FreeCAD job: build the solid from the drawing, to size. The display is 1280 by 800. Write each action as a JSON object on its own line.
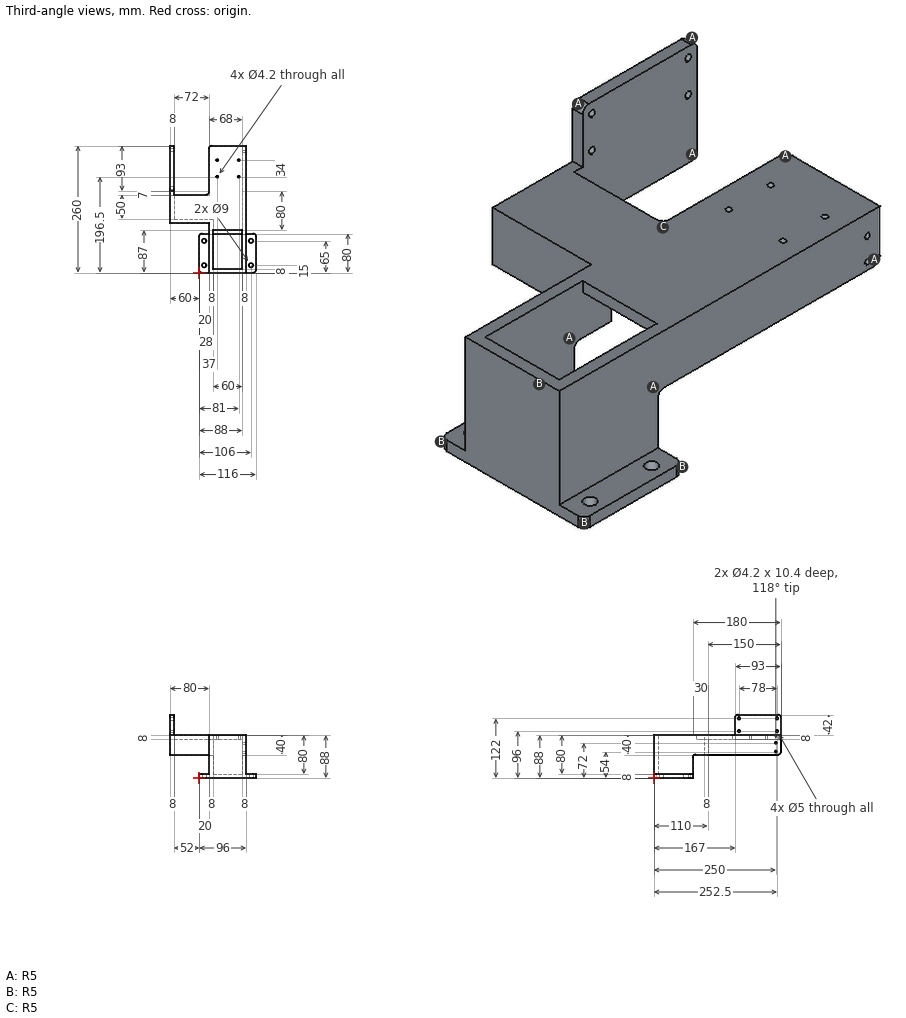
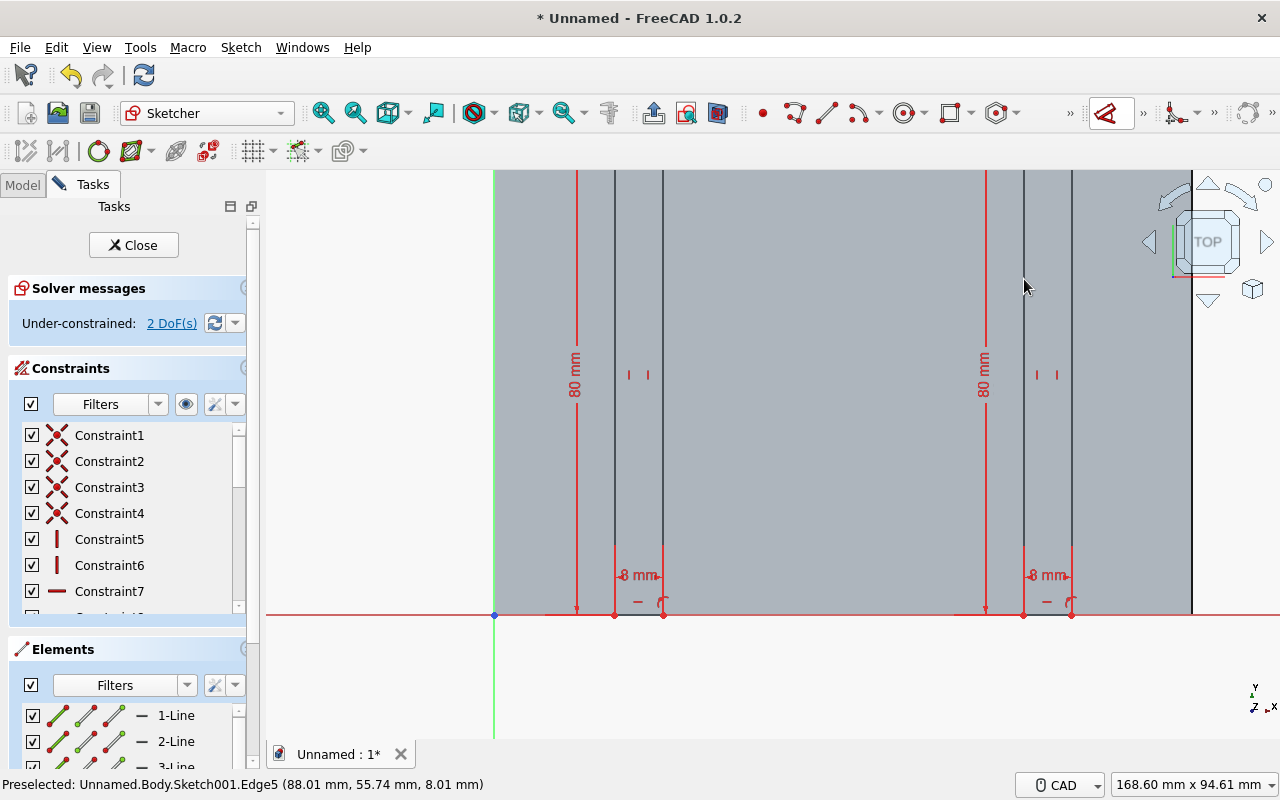
{"action": "scroll", "coordinate": [350, 711], "scroll_direction": "down", "scroll_amount": 1}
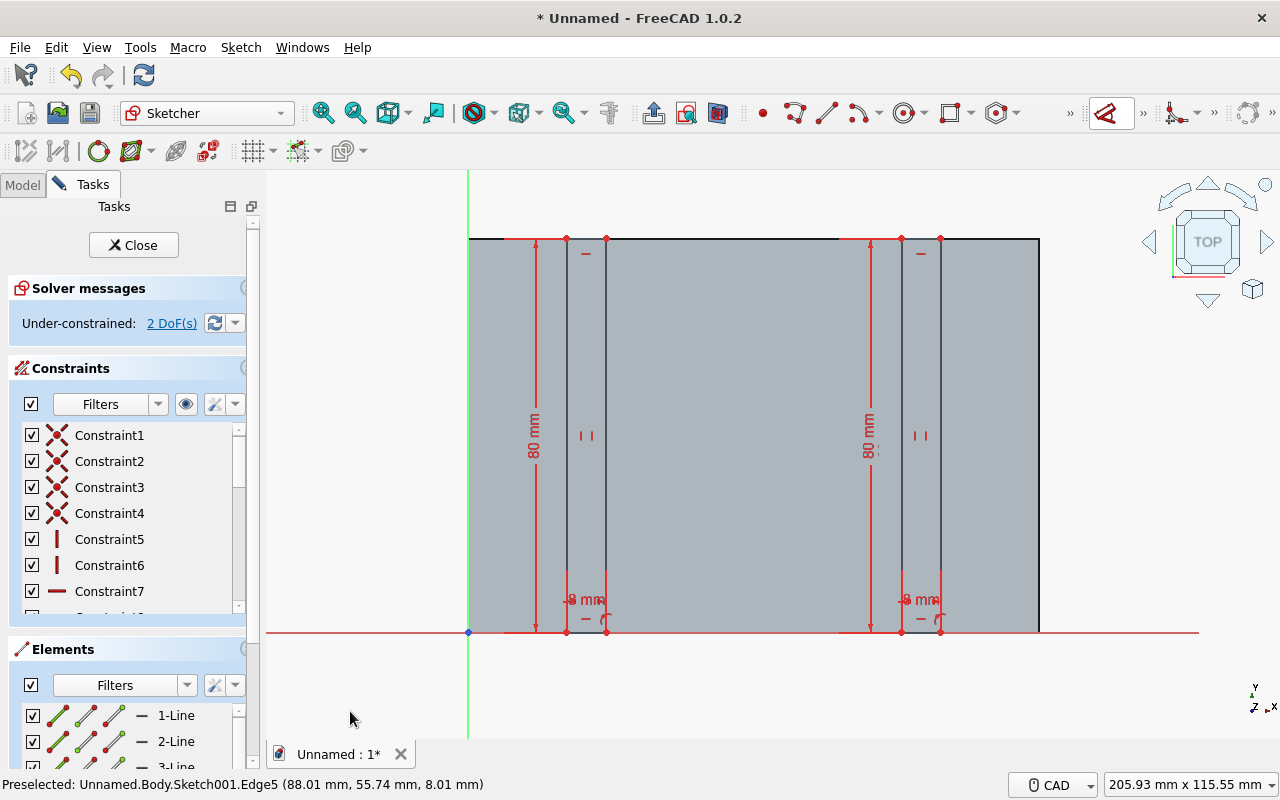
{"action": "left_click", "coordinate": [567, 239]}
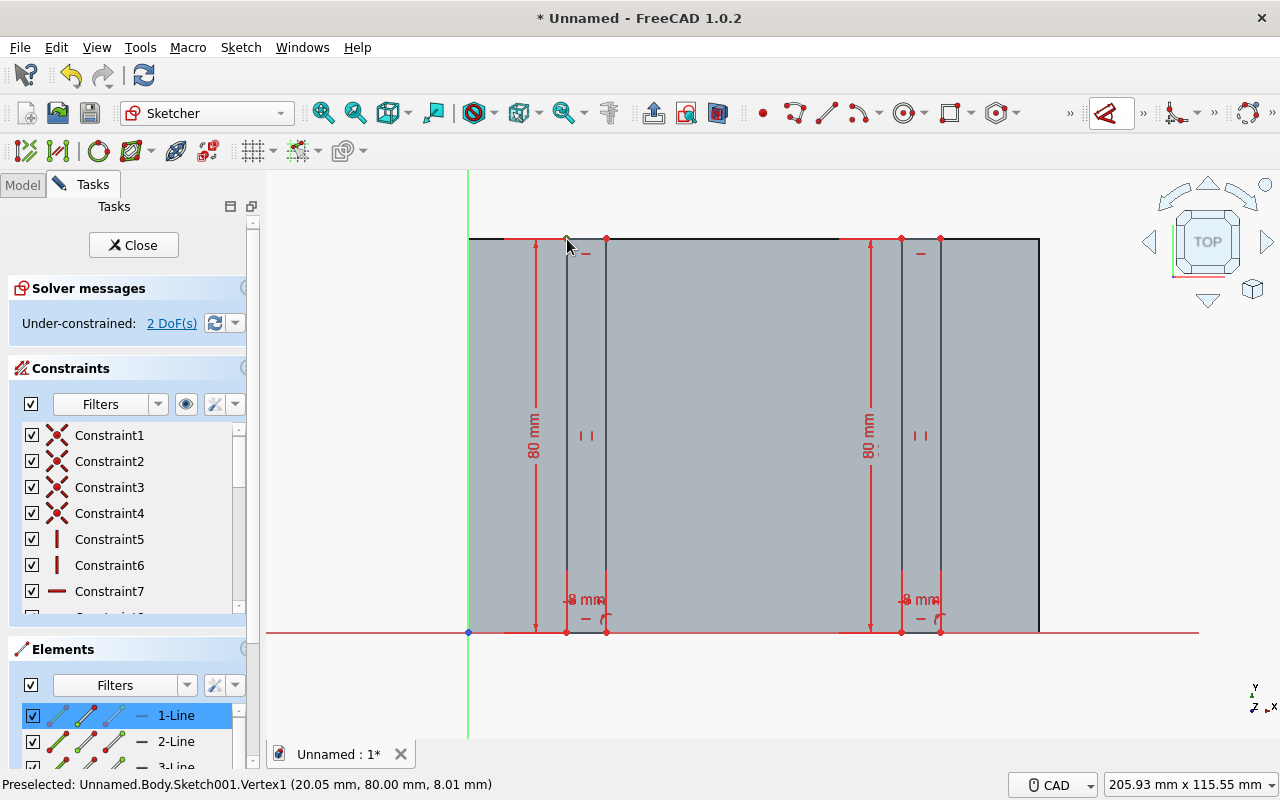
{"action": "left_click", "coordinate": [1128, 114]}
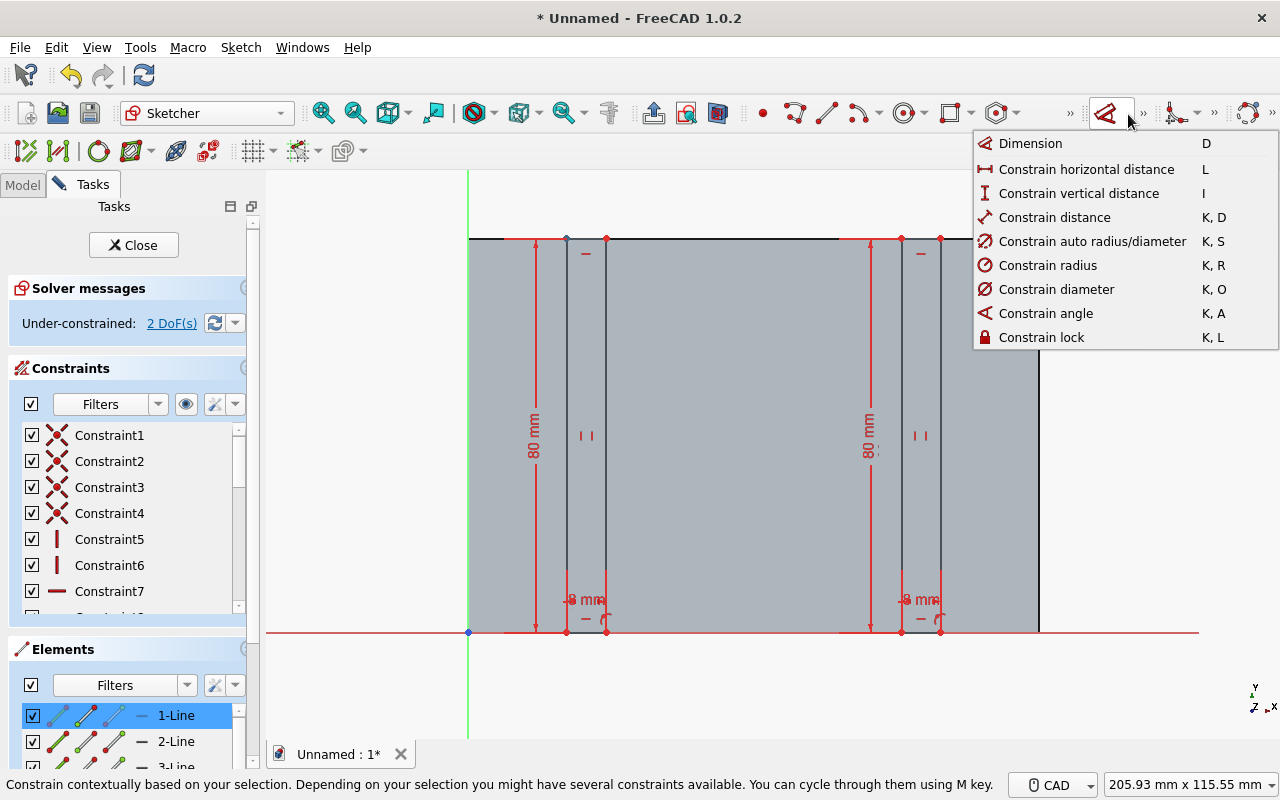
{"action": "left_click", "coordinate": [1126, 169]}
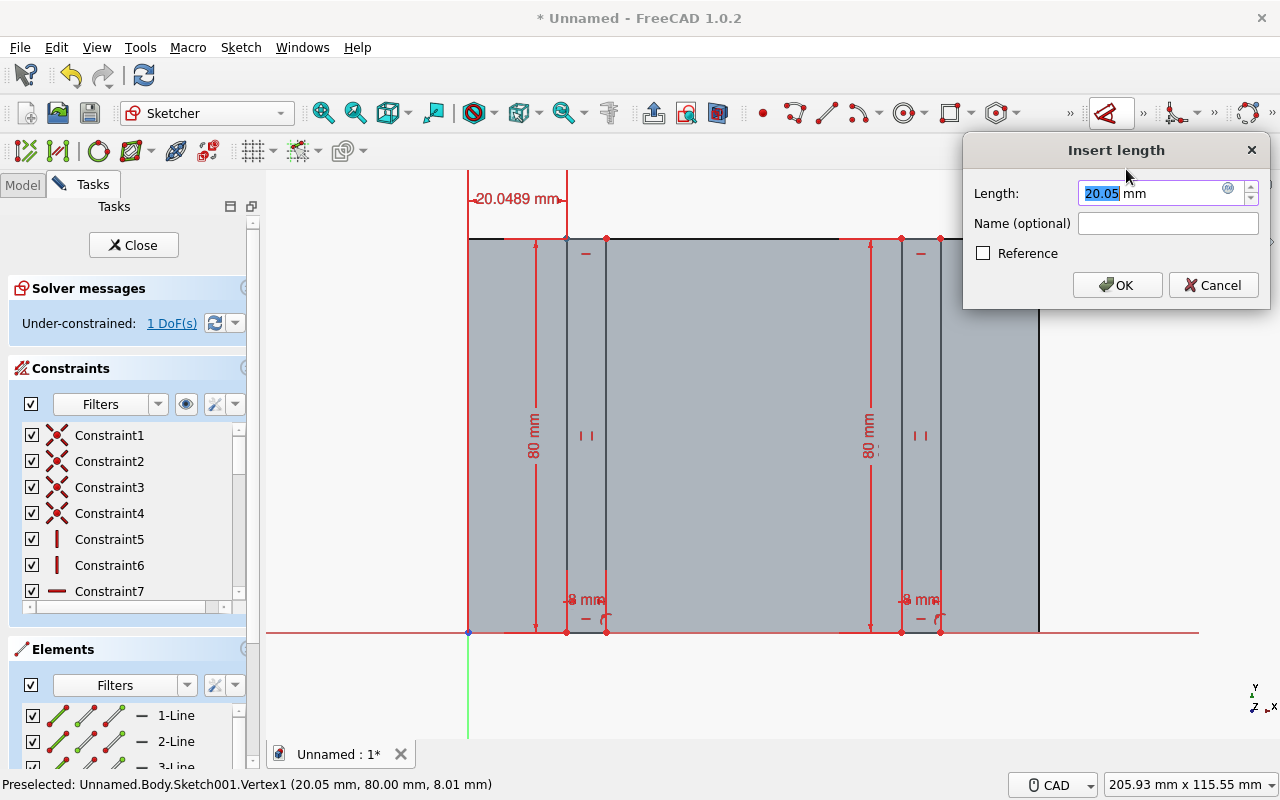
{"action": "type", "text": "20"}
{"action": "key", "text": "Return"}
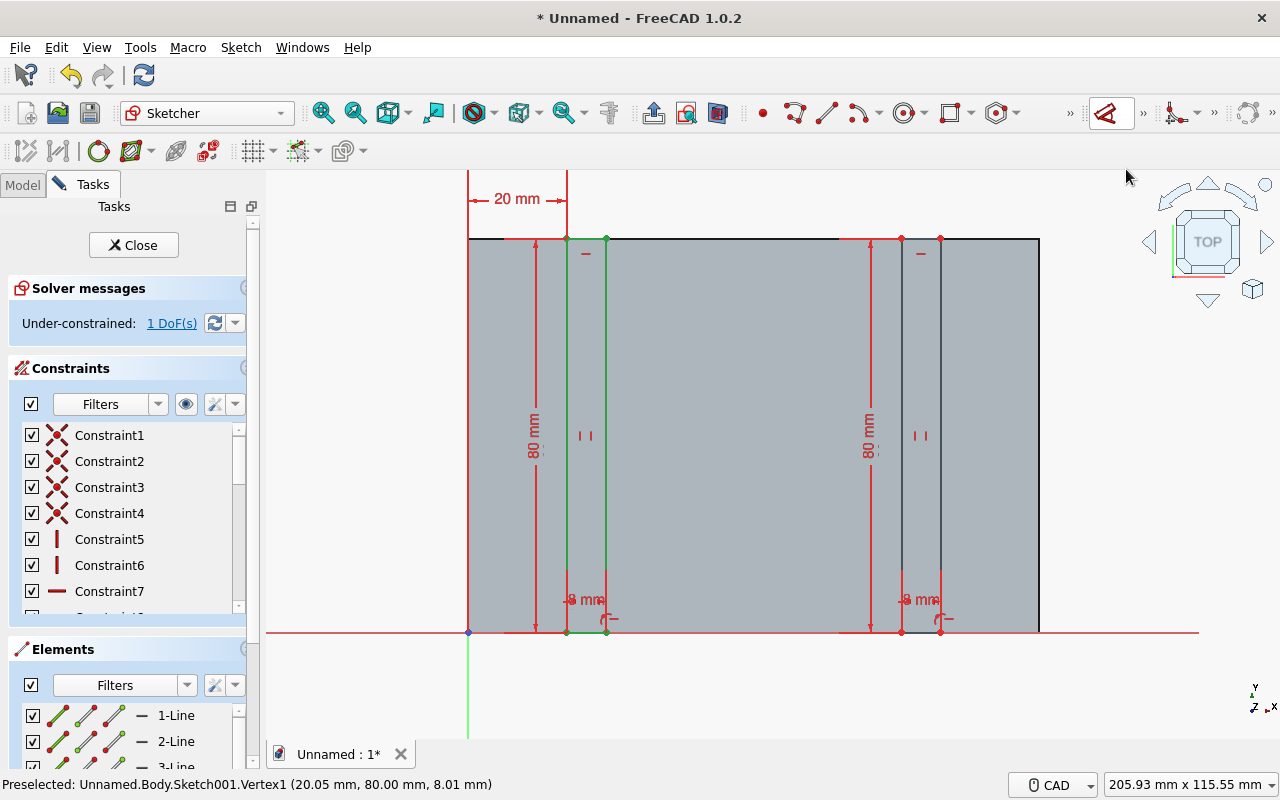
{"action": "left_click", "coordinate": [902, 239]}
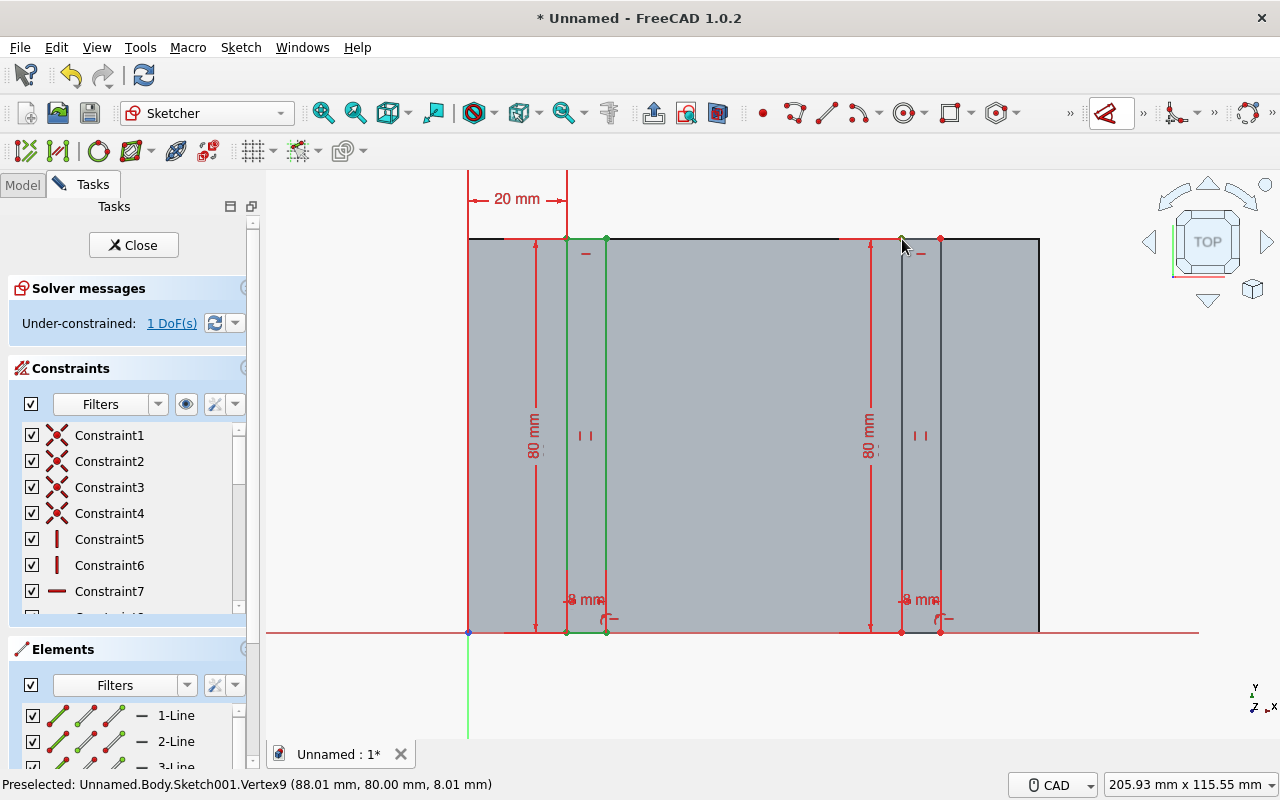
{"action": "key", "text": "l"}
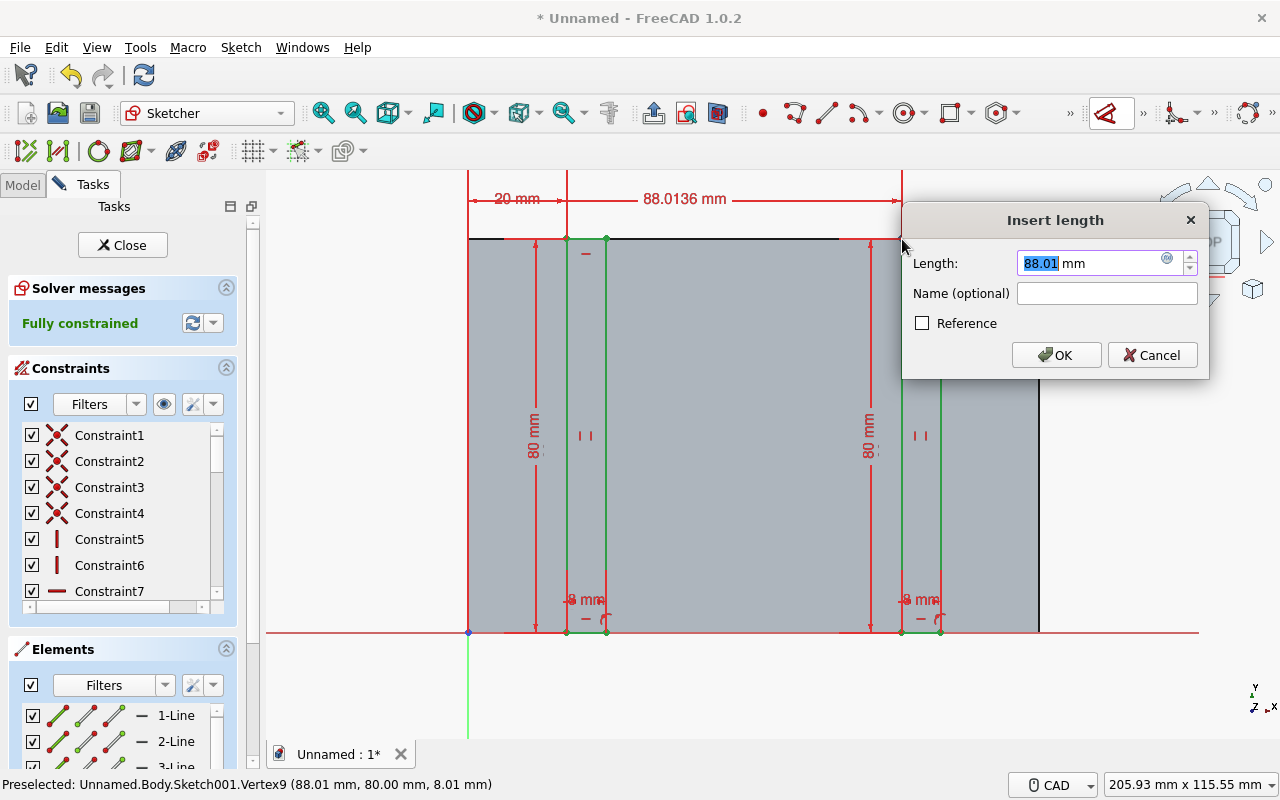
{"action": "type", "text": "88"}
{"action": "key", "text": "Return"}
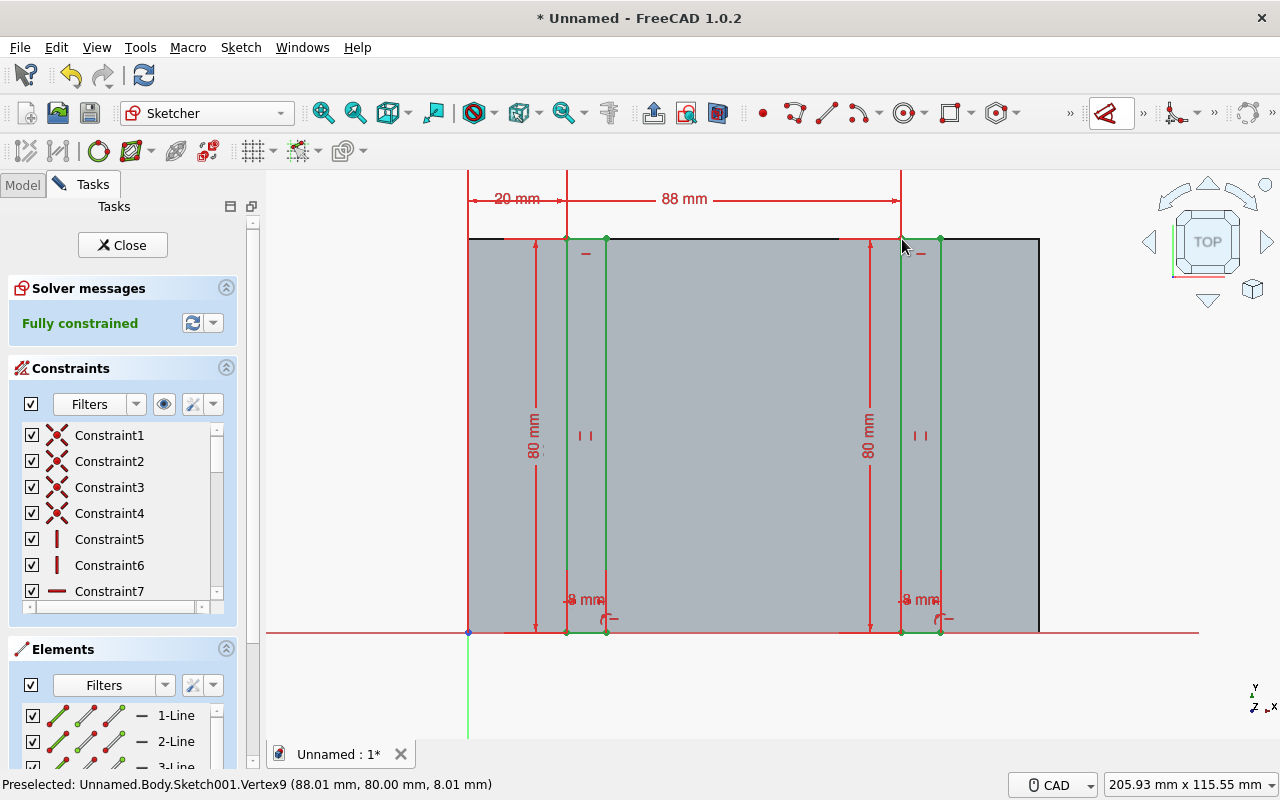
{"action": "left_click", "coordinate": [123, 245]}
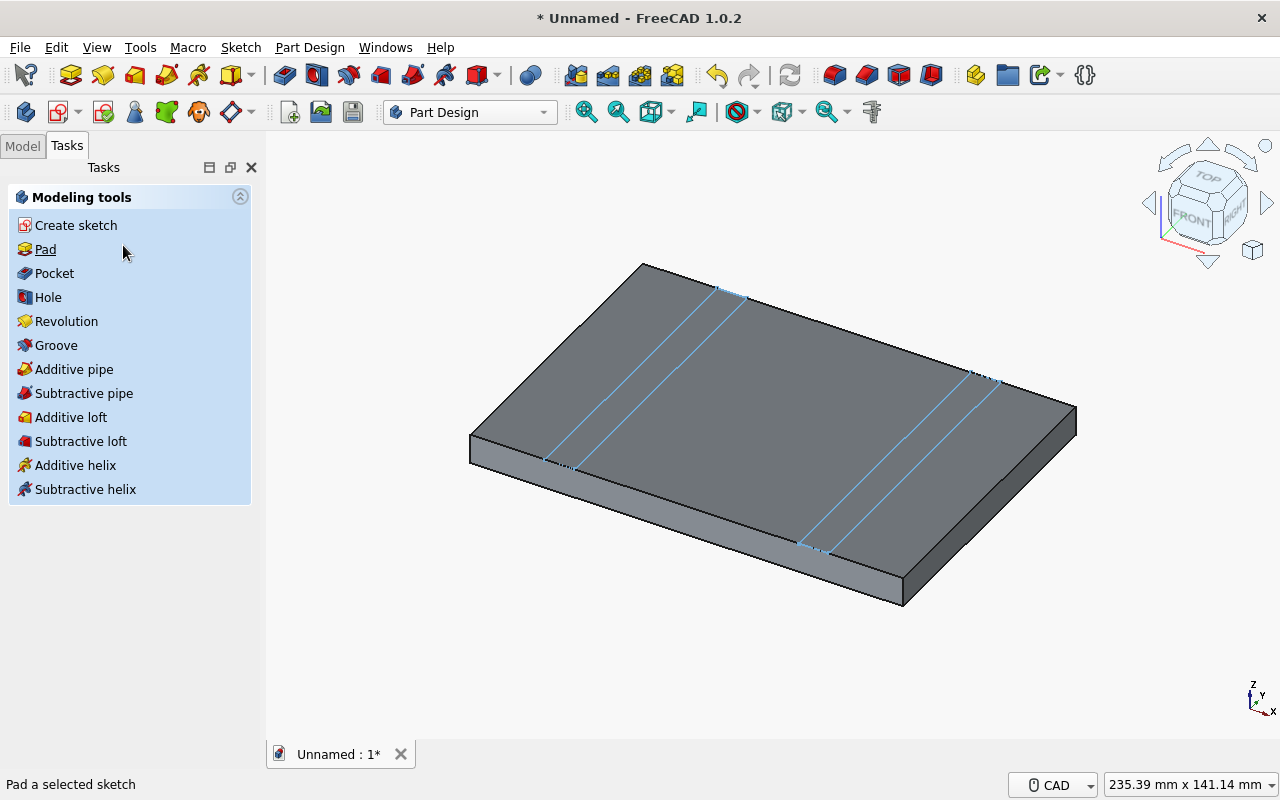
{"action": "left_click", "coordinate": [72, 76]}